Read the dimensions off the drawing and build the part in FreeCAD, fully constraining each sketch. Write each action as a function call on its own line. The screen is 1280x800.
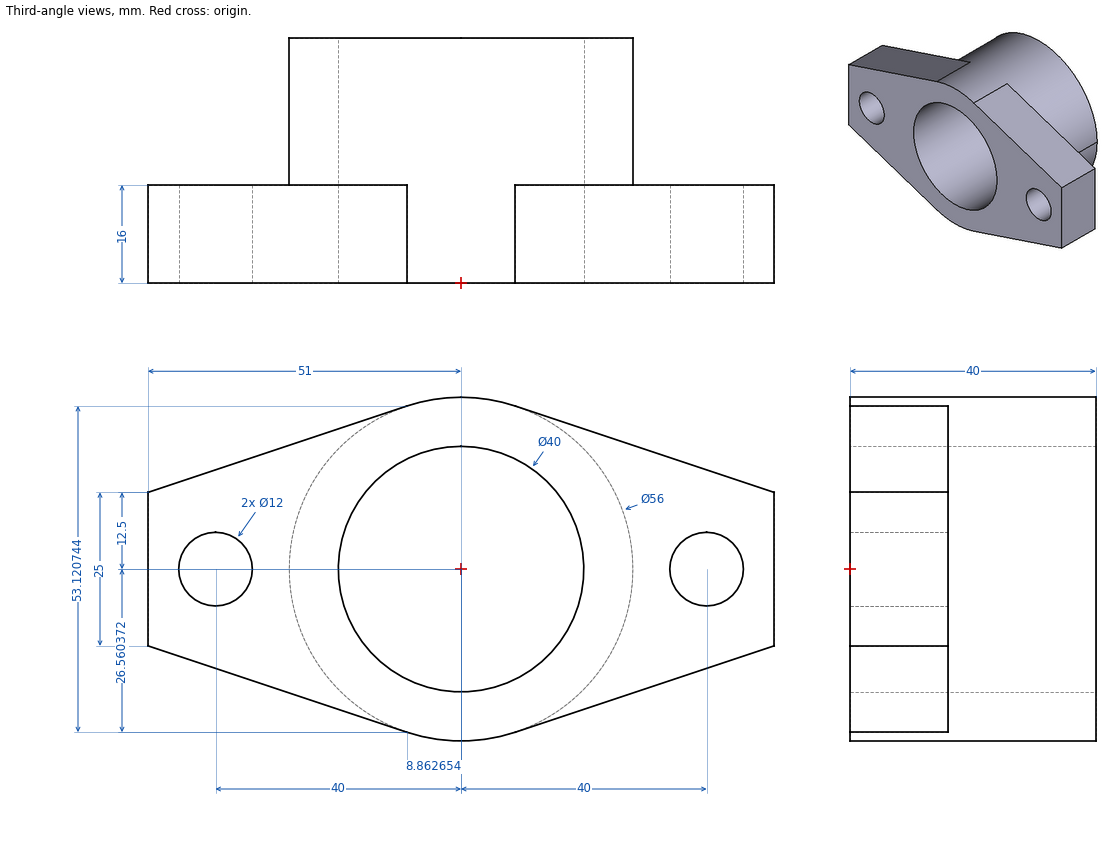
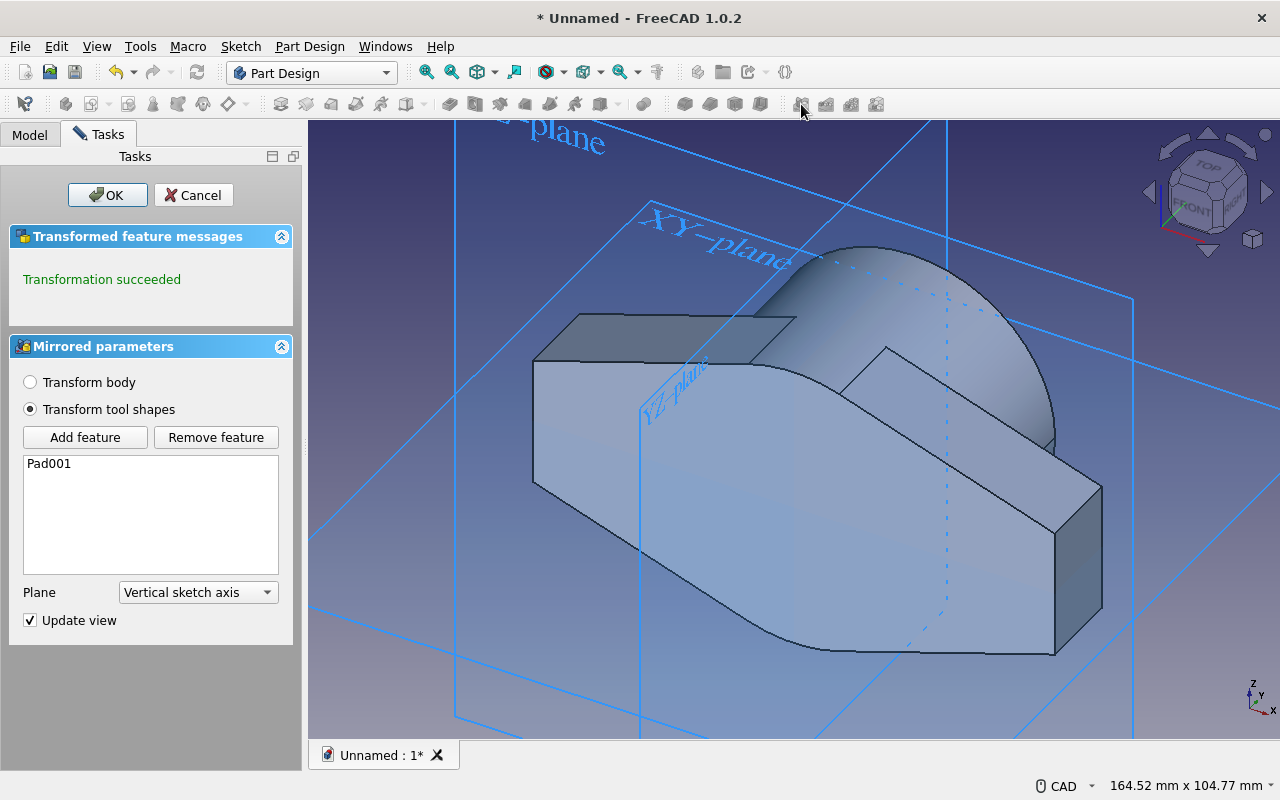
click(199, 592)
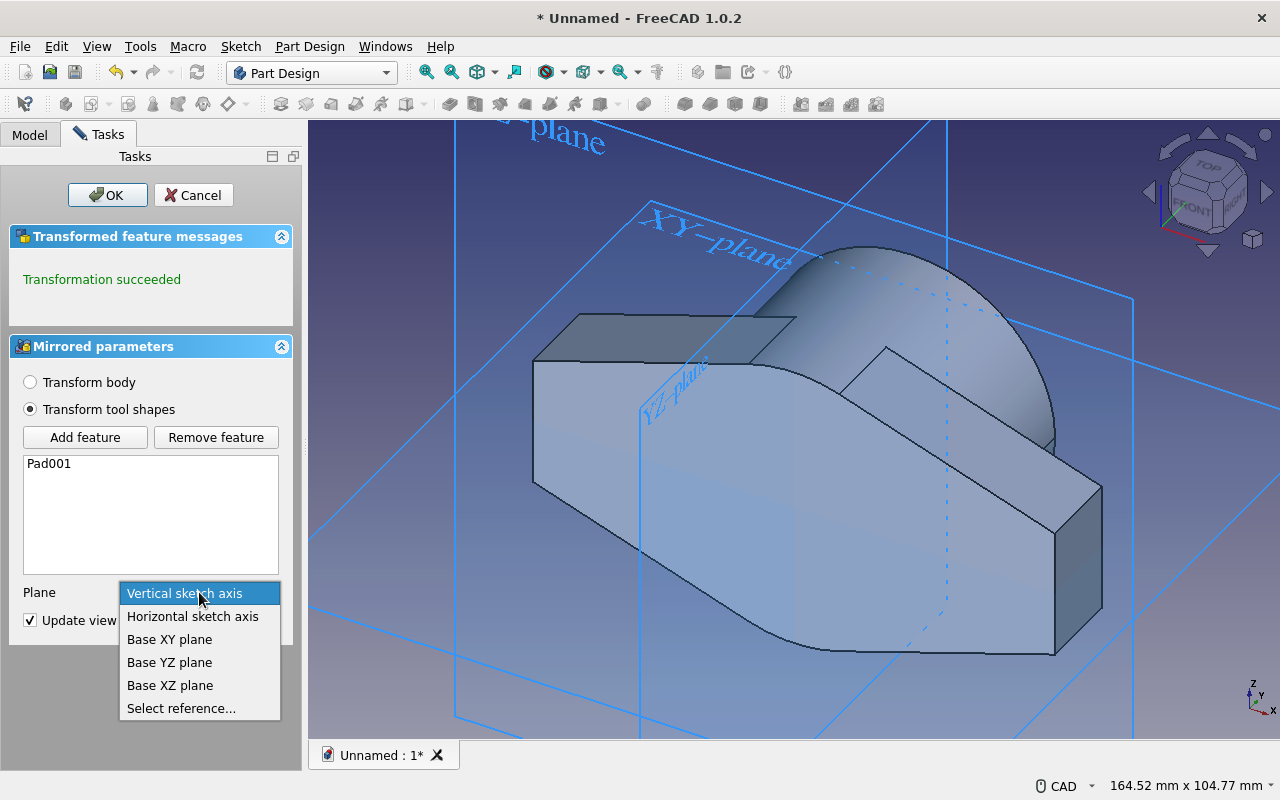
click(198, 662)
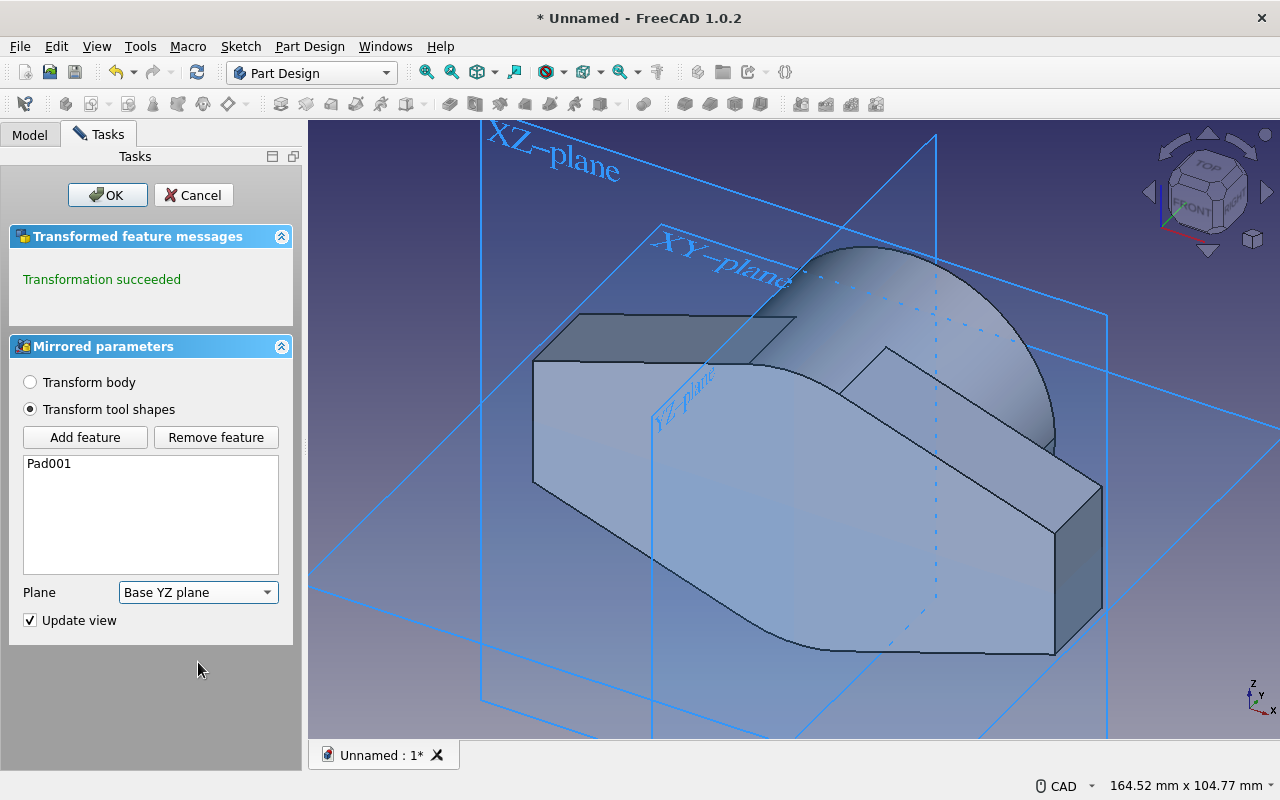
click(108, 195)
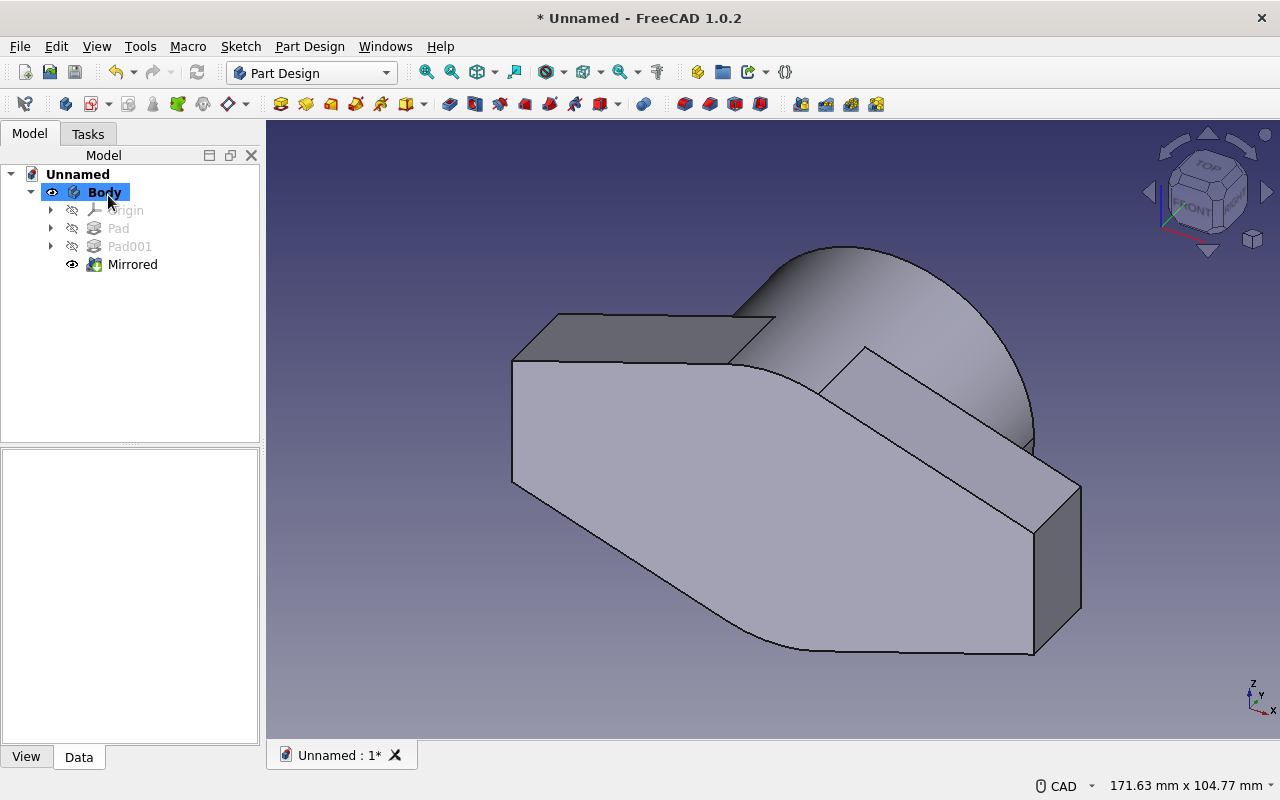
key(4)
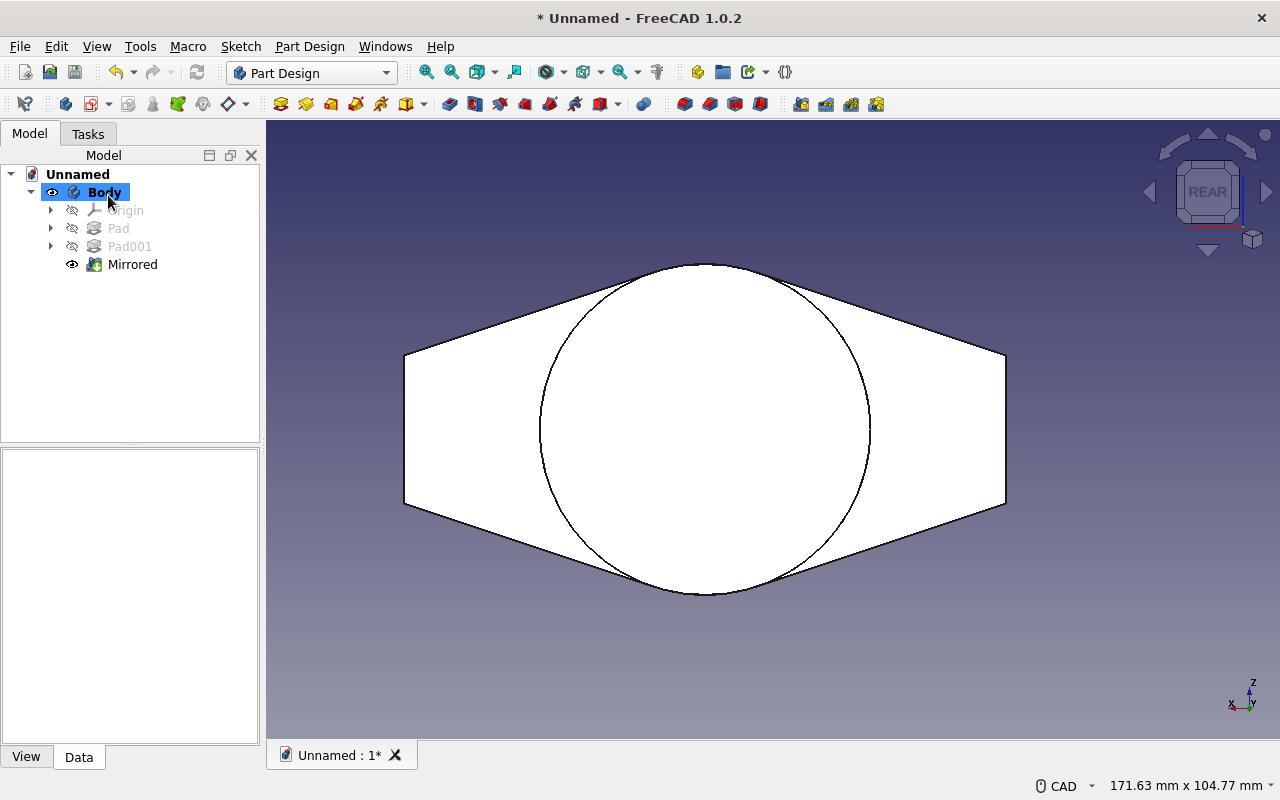
click(705, 429)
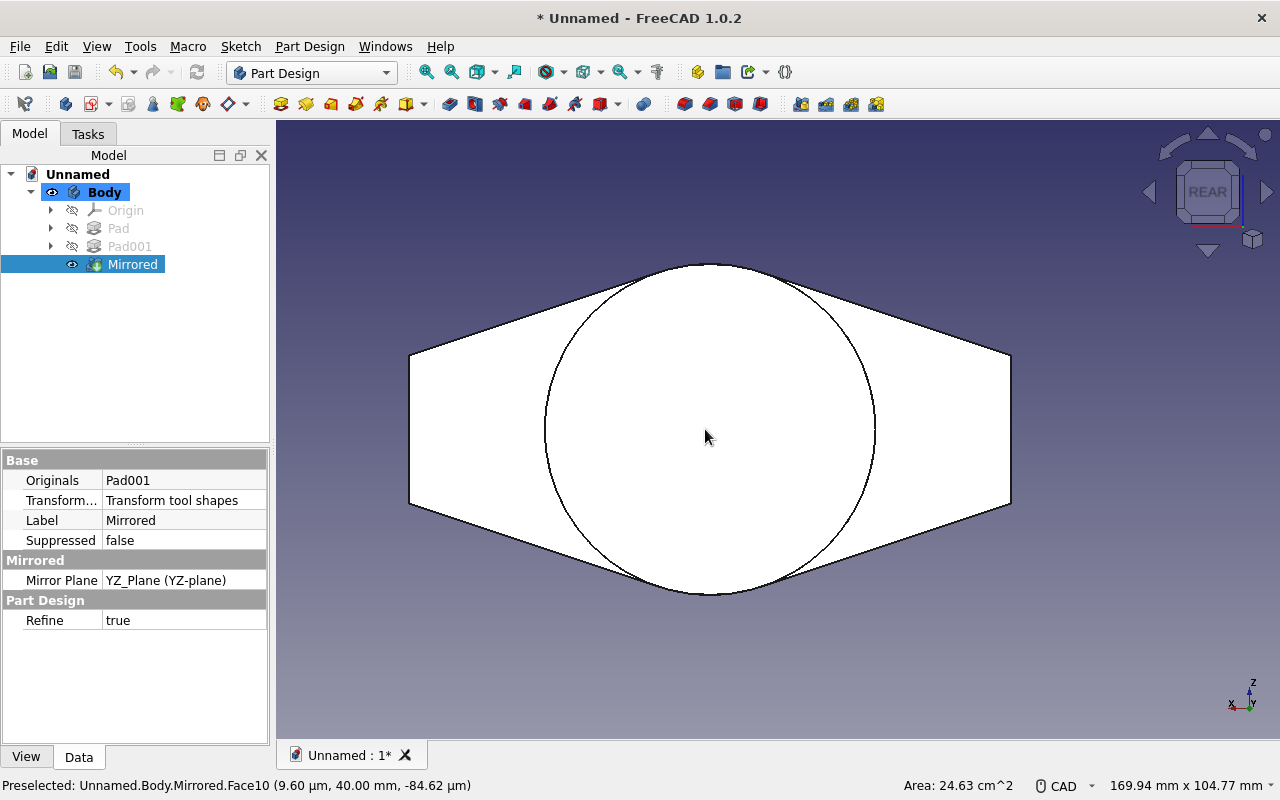
click(90, 104)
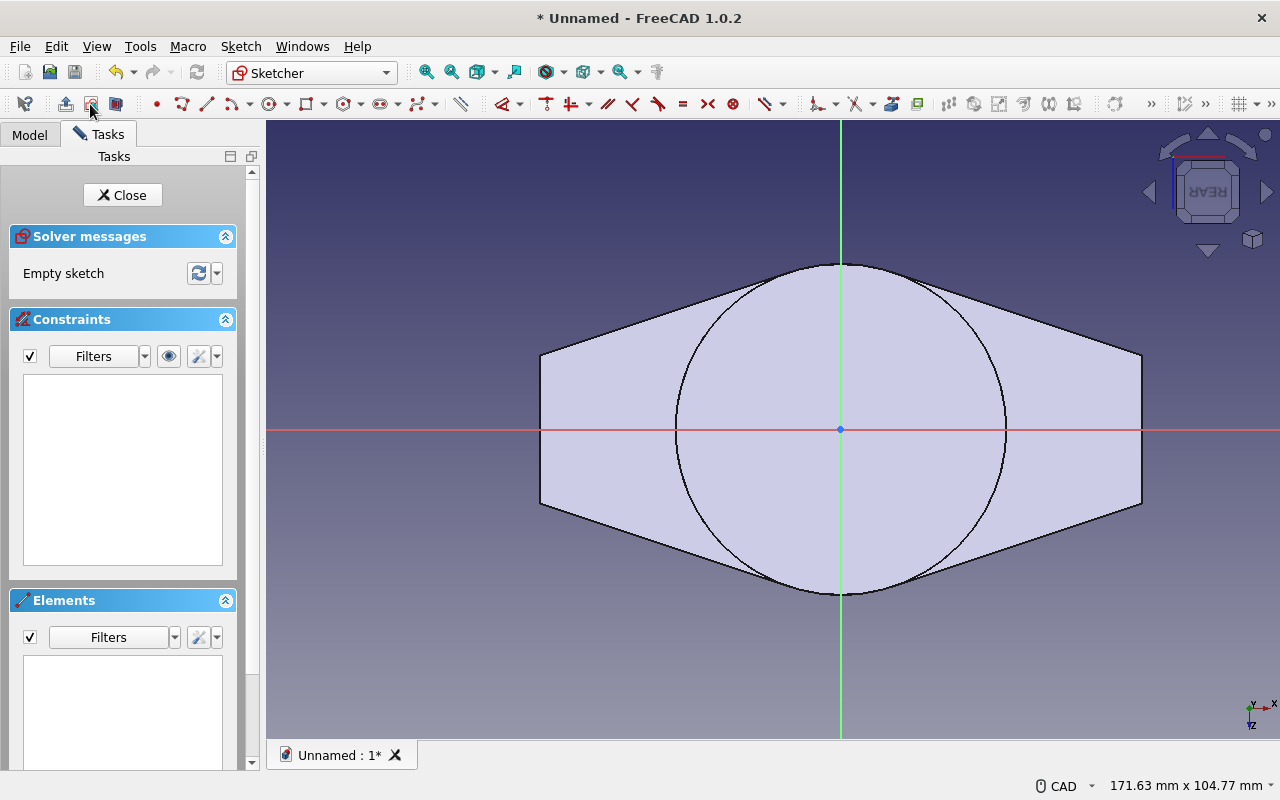
scroll(1007, 429, up, 3)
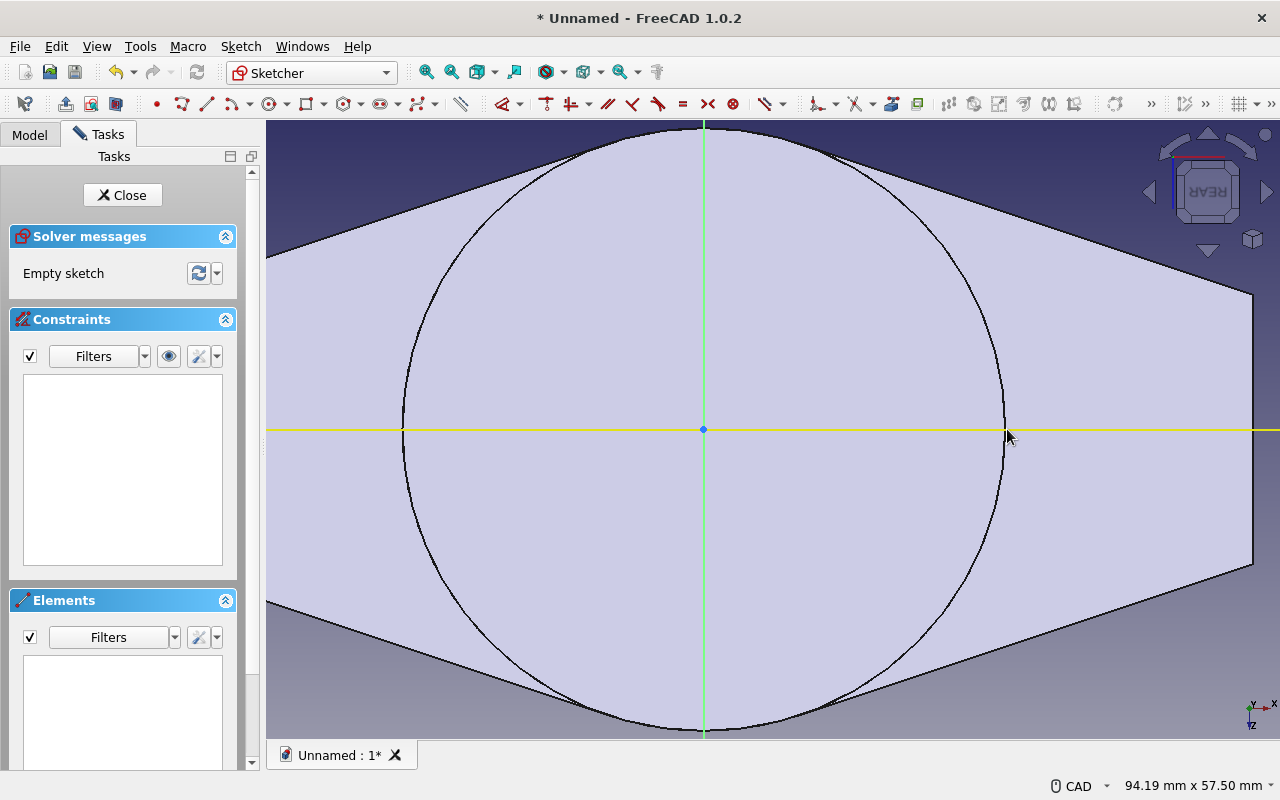
click(268, 104)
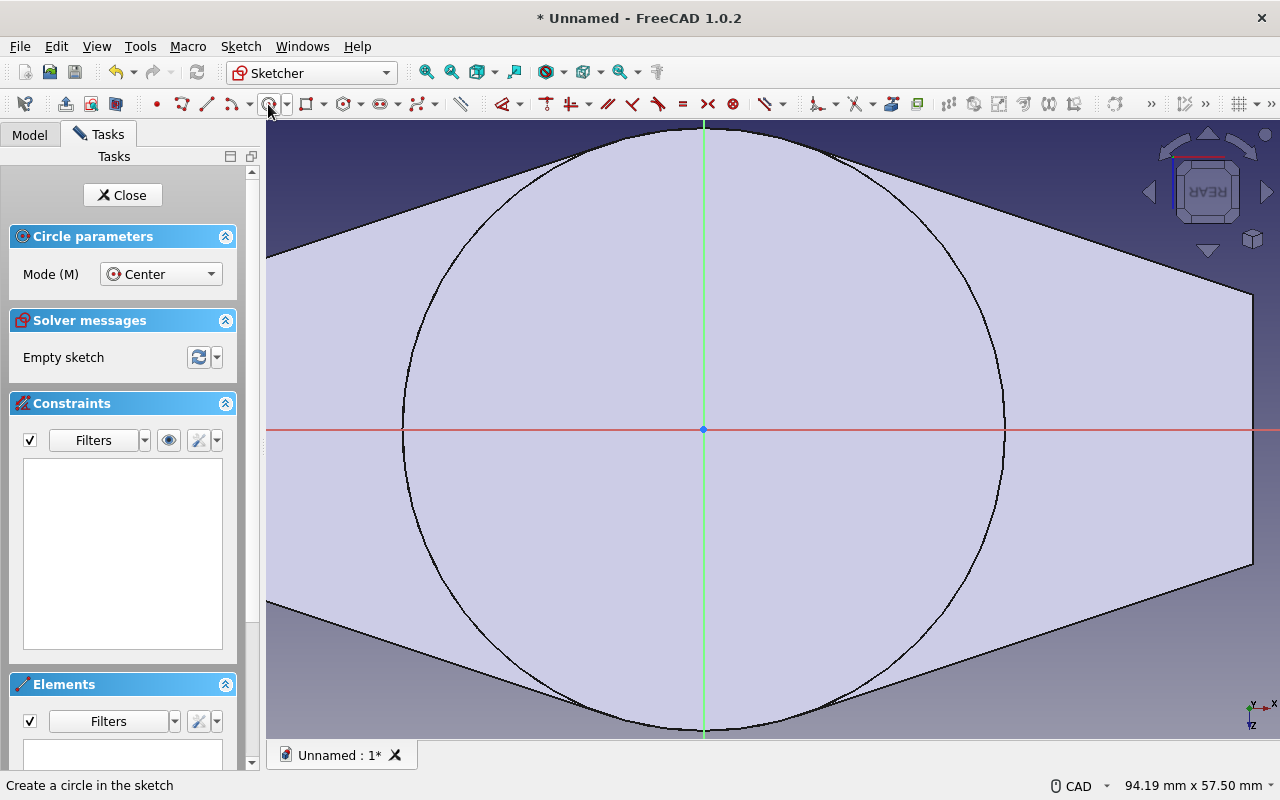
click(704, 429)
move(856, 277)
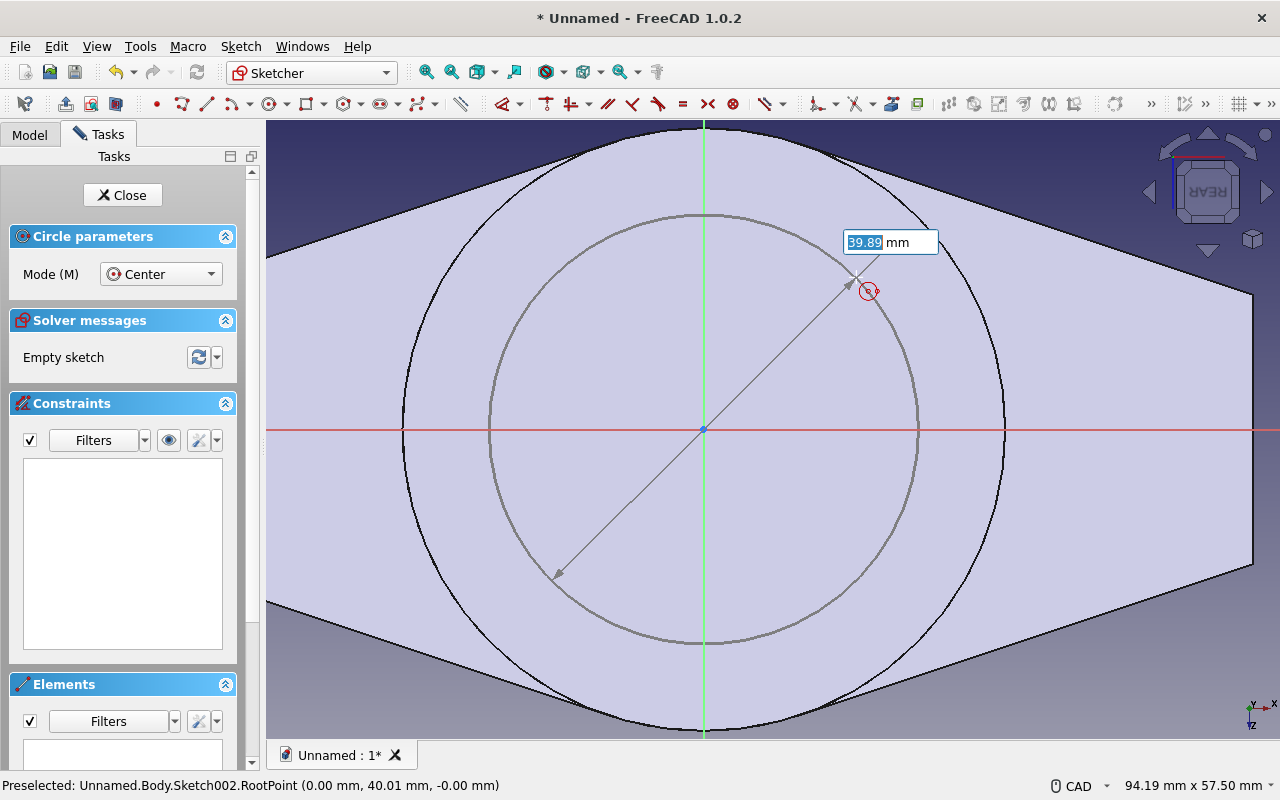
text(40)
key(Return)
key(Escape)